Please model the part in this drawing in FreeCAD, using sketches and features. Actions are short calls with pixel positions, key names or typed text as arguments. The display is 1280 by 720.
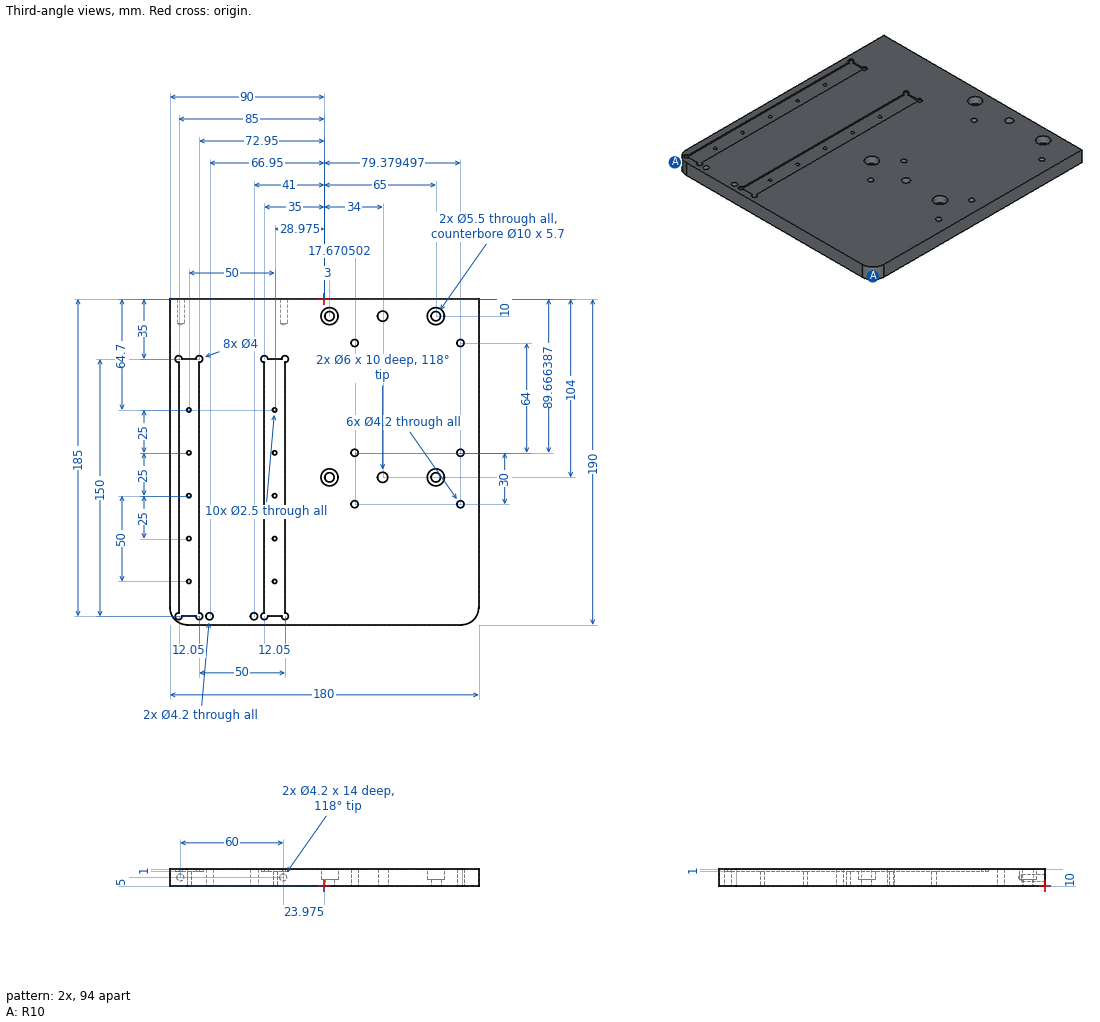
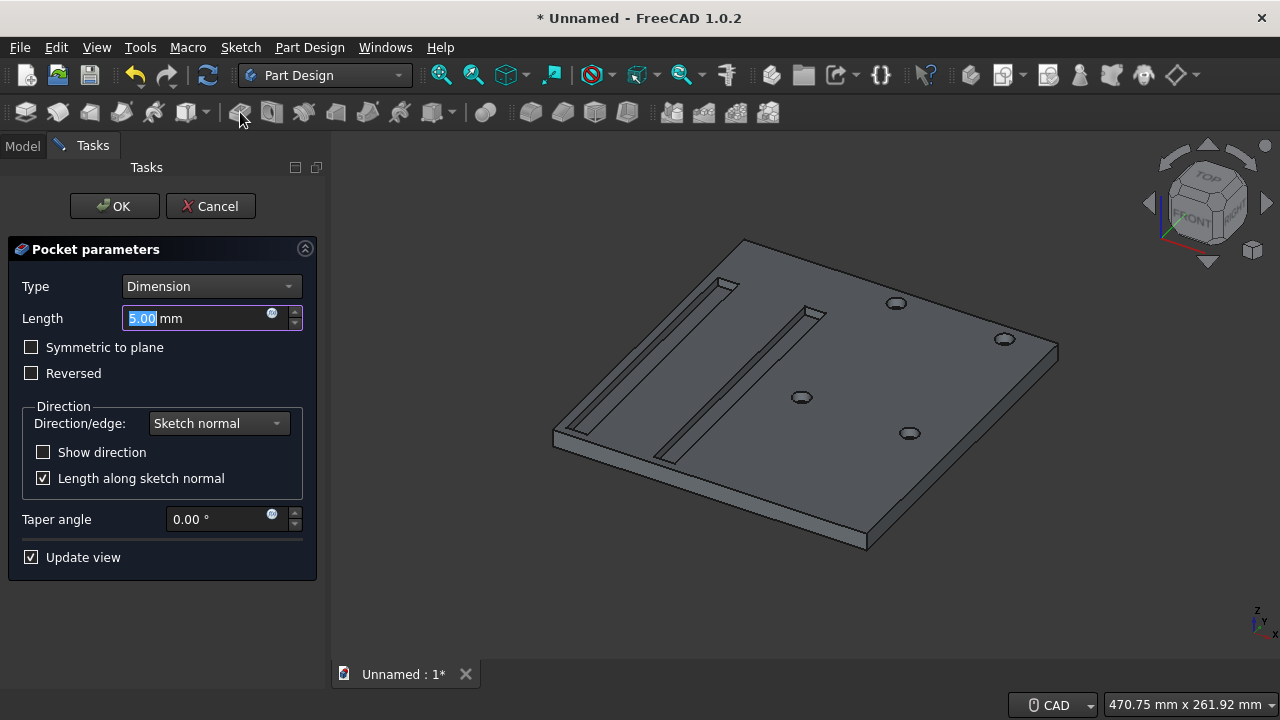
text(1)
key(Tab)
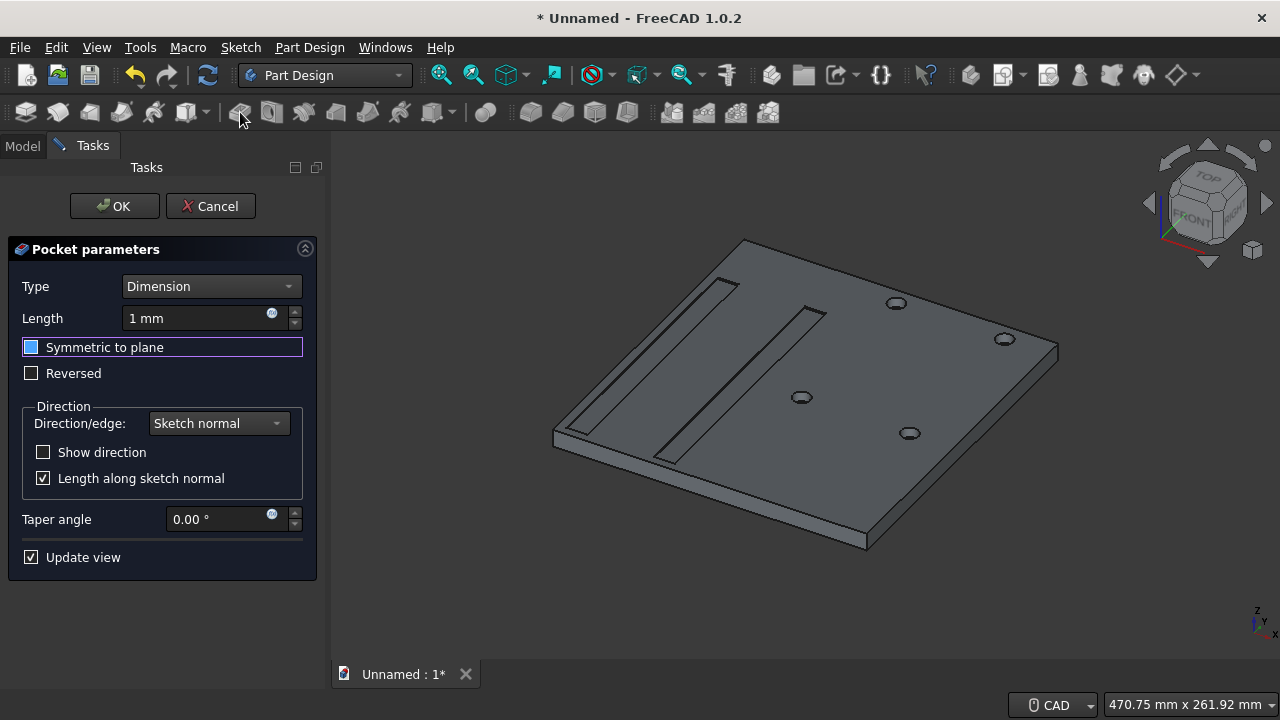
click(115, 206)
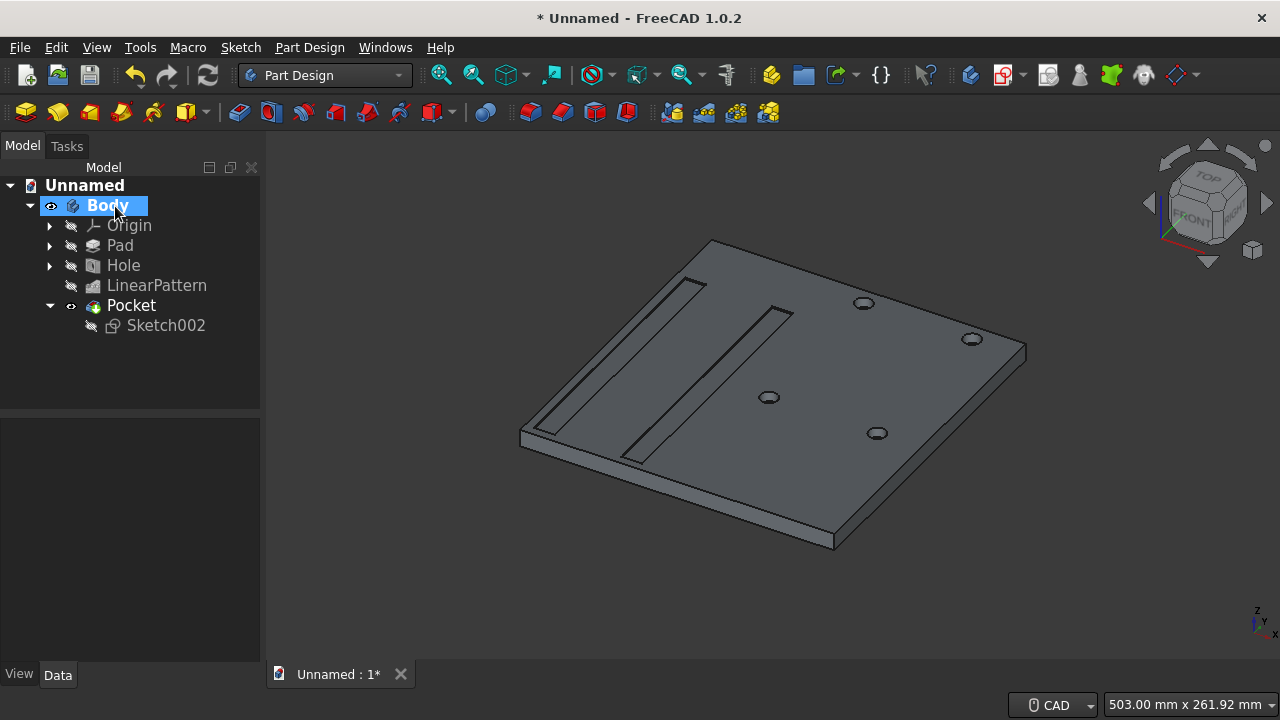
click(763, 455)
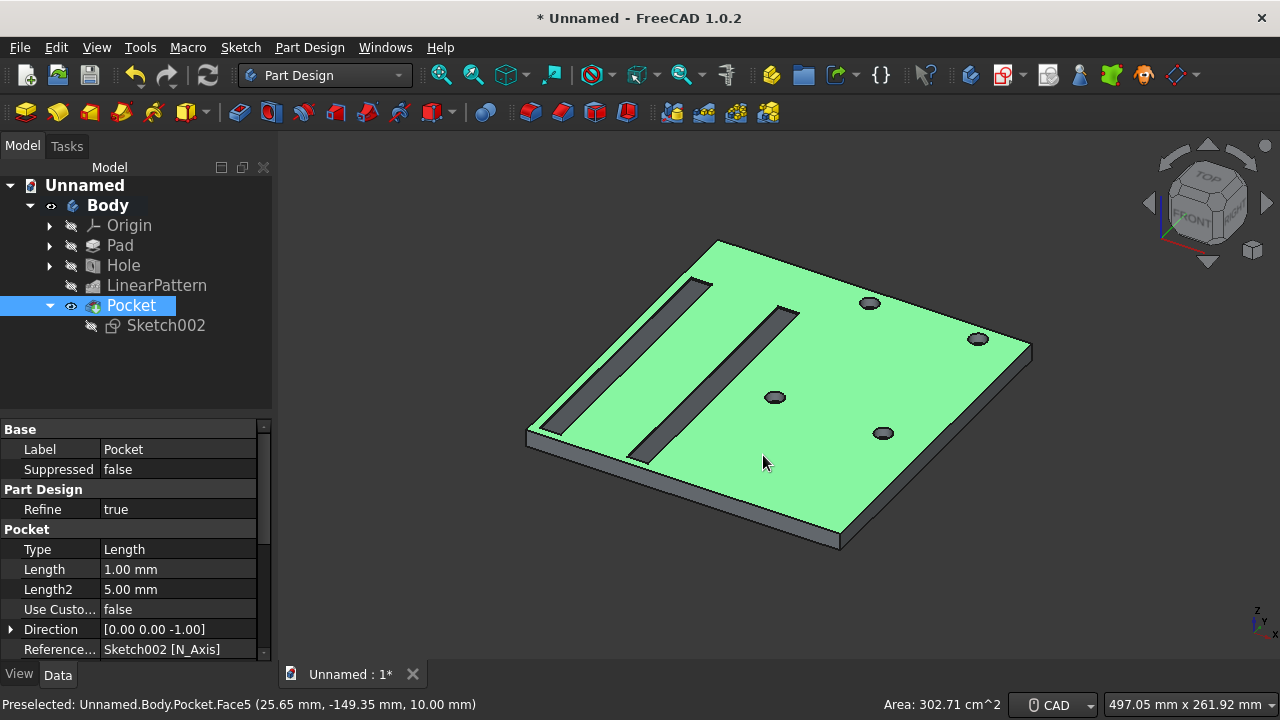
click(1004, 76)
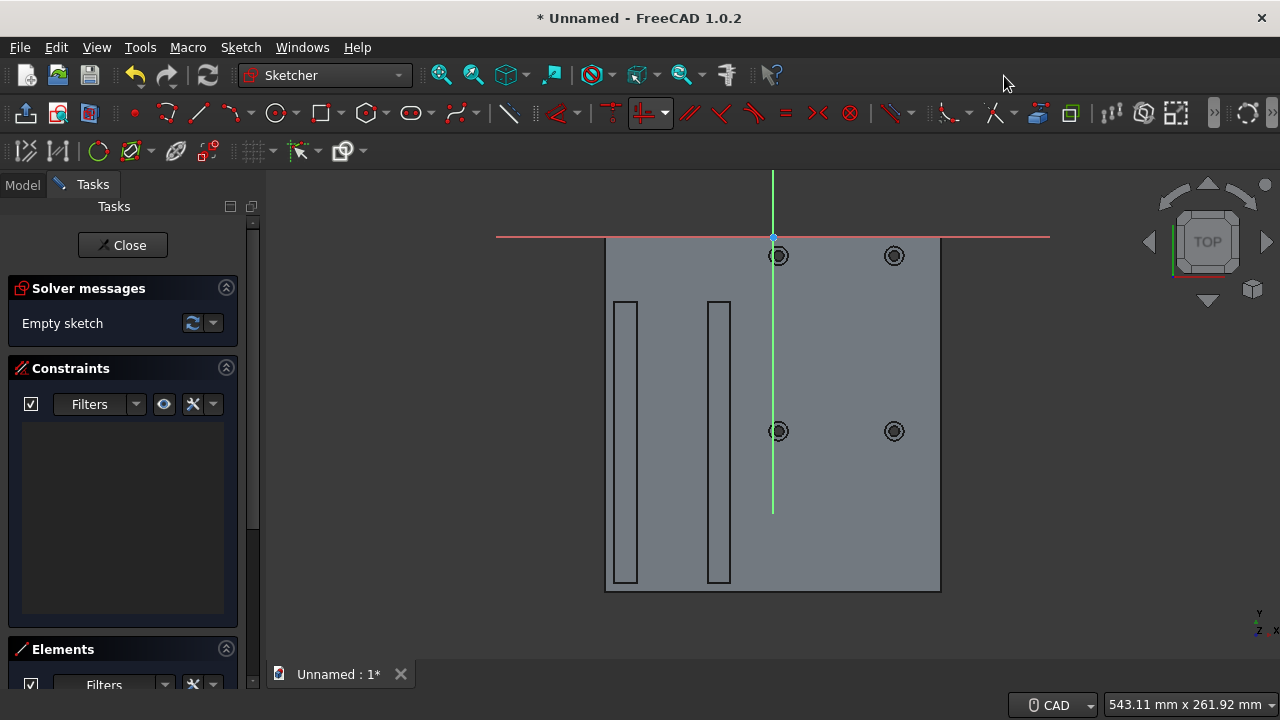
key(g)
key(c)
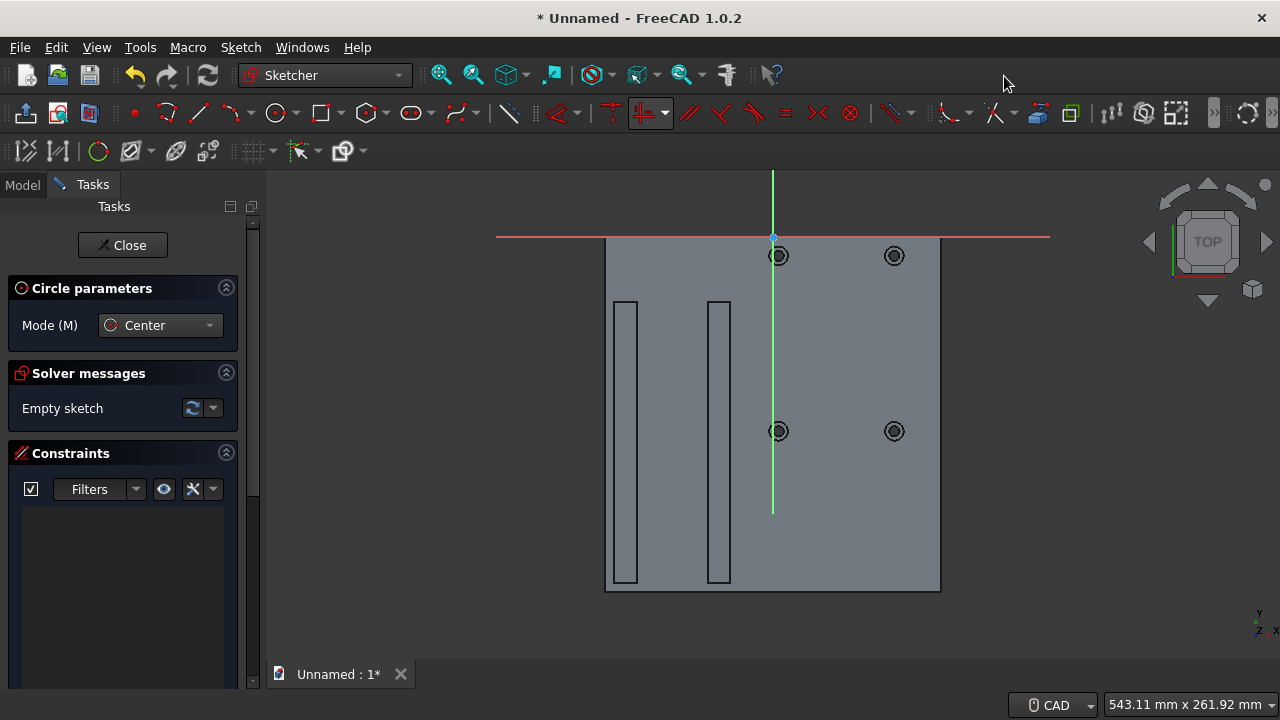
scroll(637, 302, up, 10)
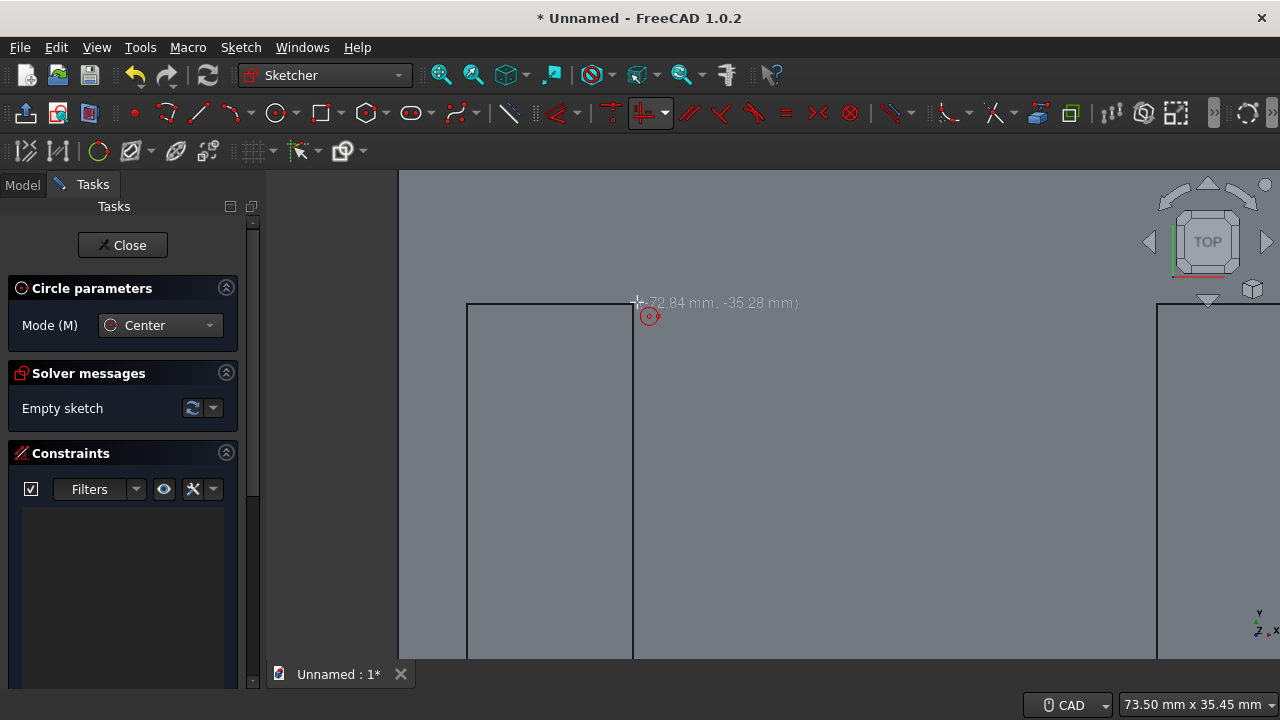
scroll(663, 328, down, 11)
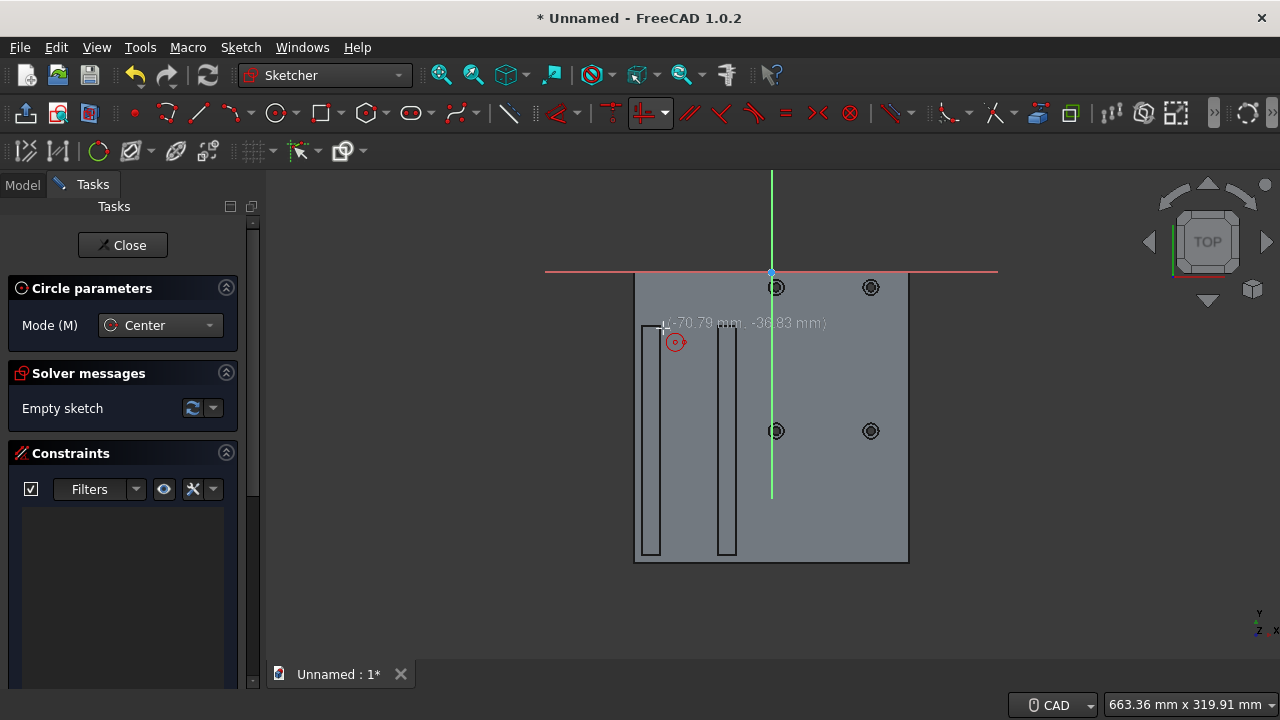
click(660, 326)
move(662, 323)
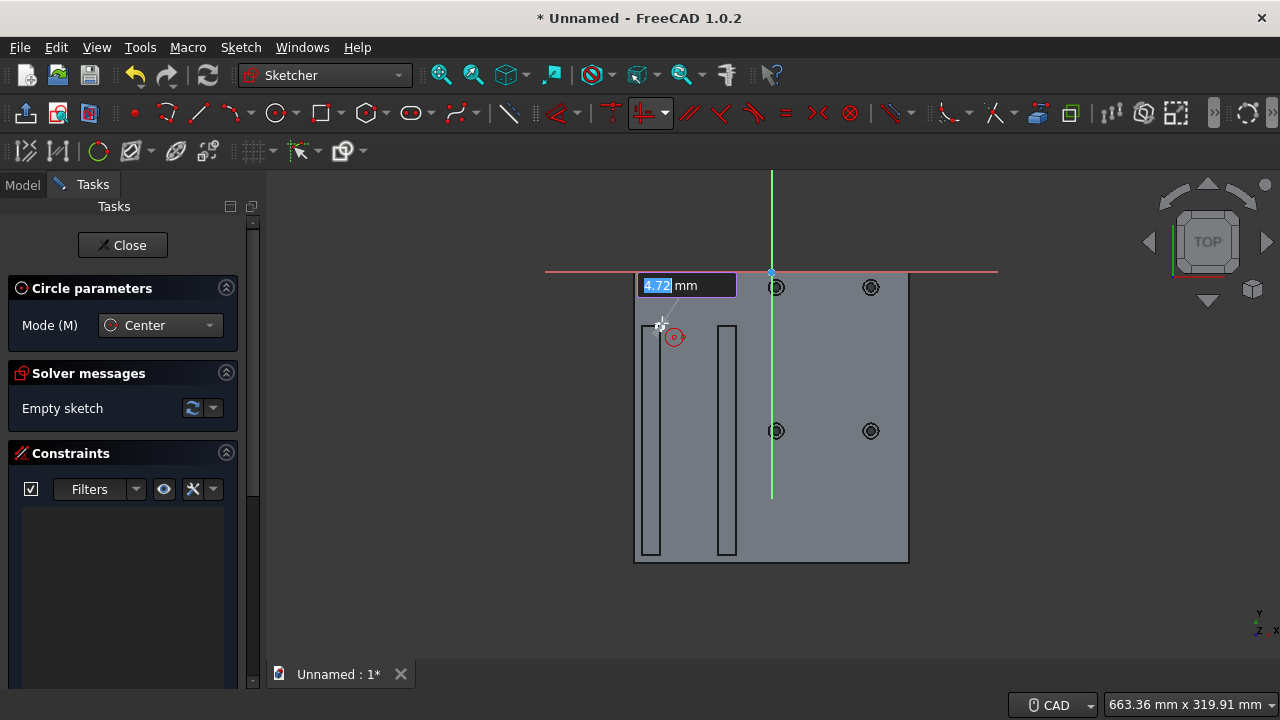
text(4)
key(Return)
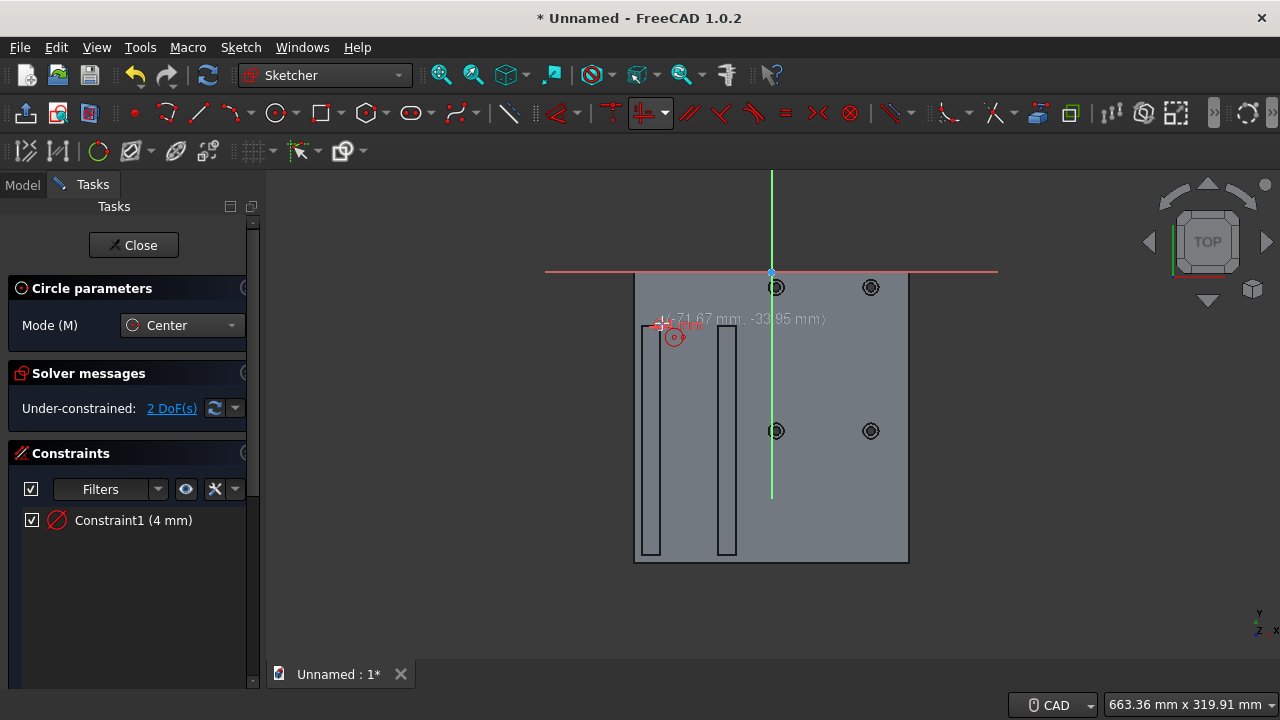
scroll(642, 326, up, 11)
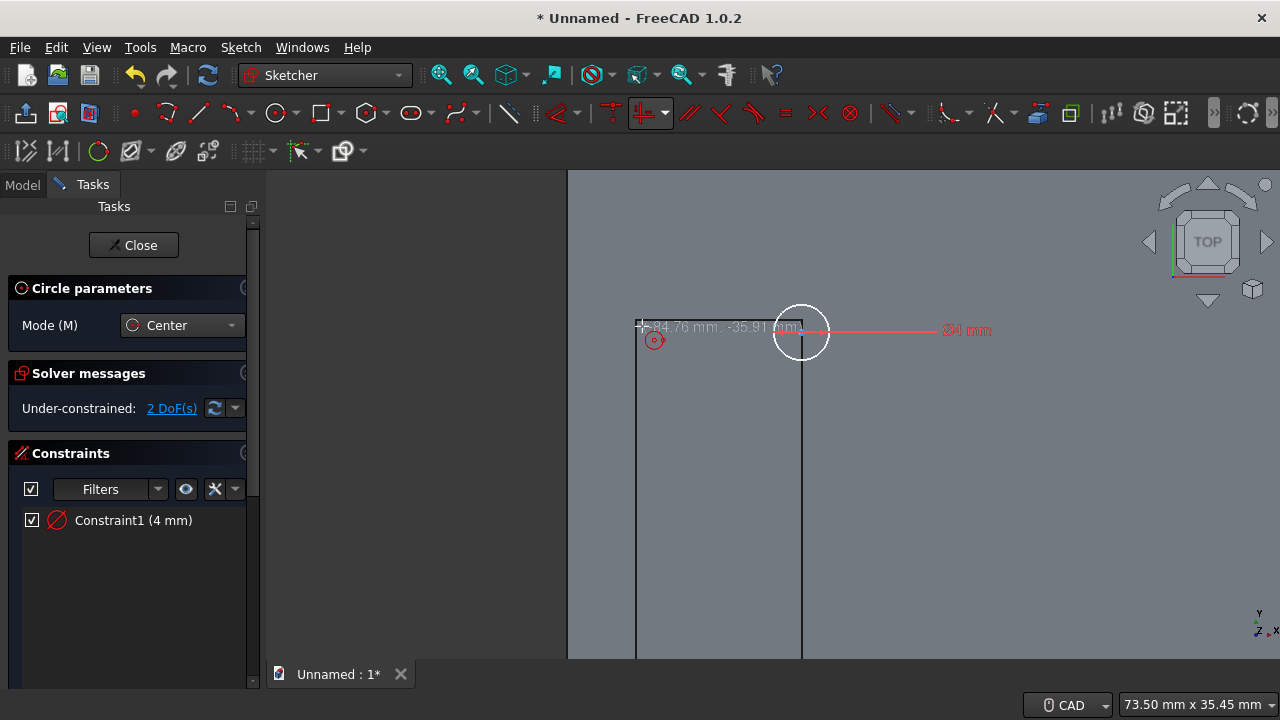
scroll(642, 326, down, 11)